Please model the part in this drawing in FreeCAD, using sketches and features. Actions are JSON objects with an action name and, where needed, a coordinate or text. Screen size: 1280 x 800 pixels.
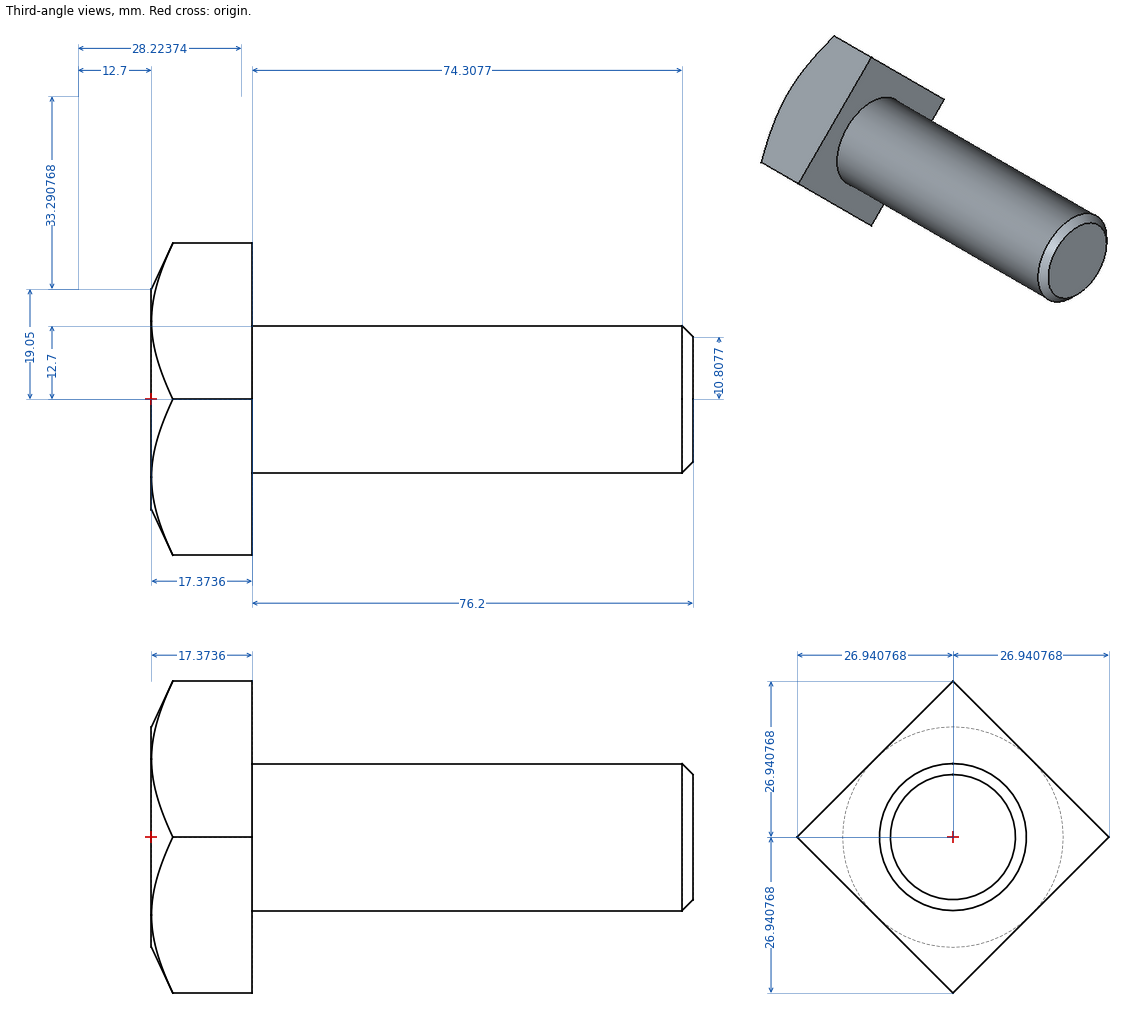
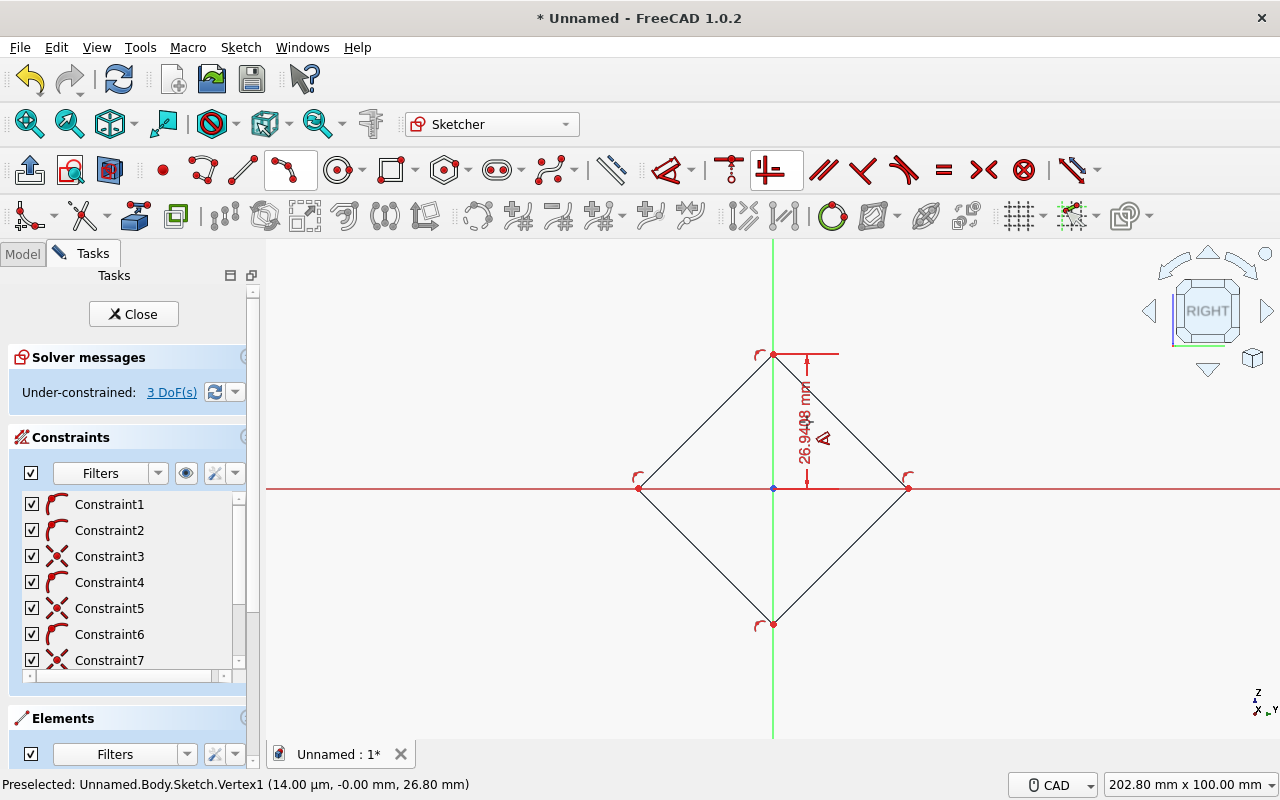
{"action": "left_click", "coordinate": [638, 489]}
{"action": "left_click", "coordinate": [705, 523]}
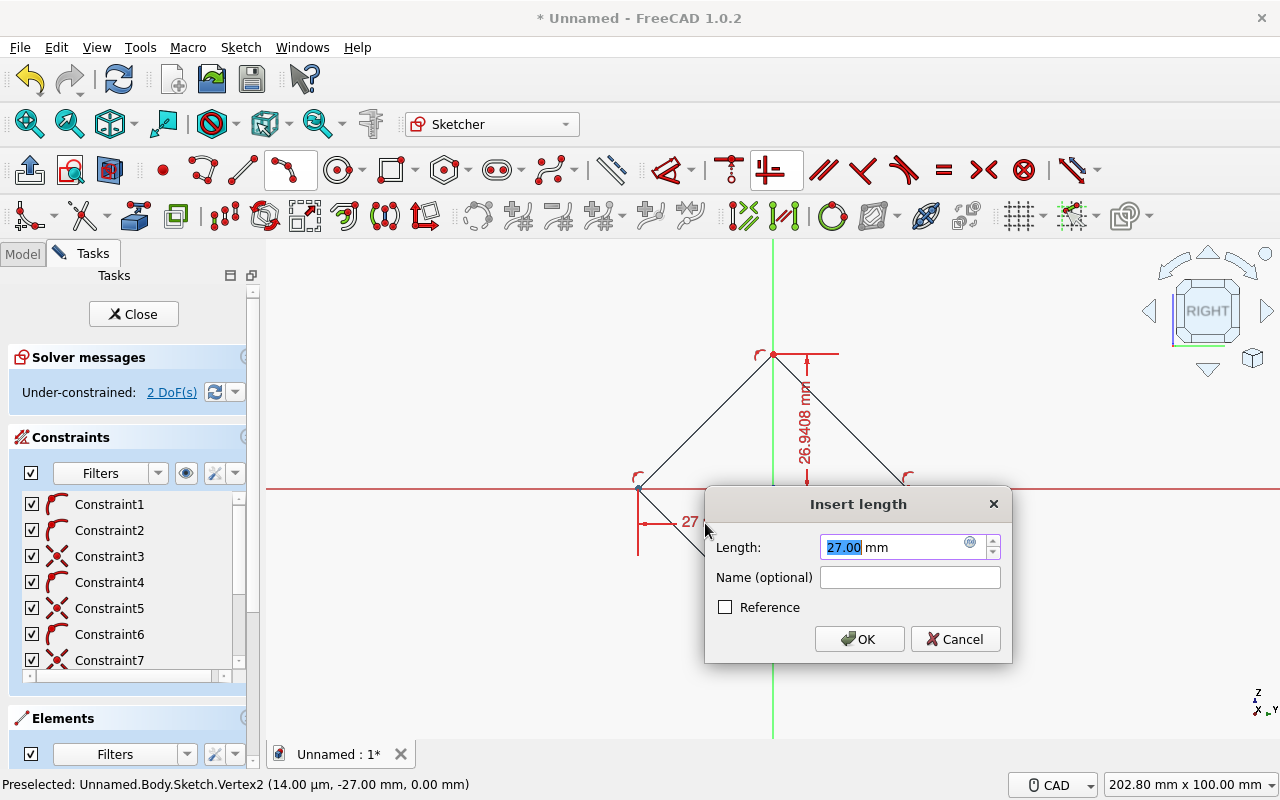
{"action": "type", "text": "26.940768"}
{"action": "key", "text": "Return"}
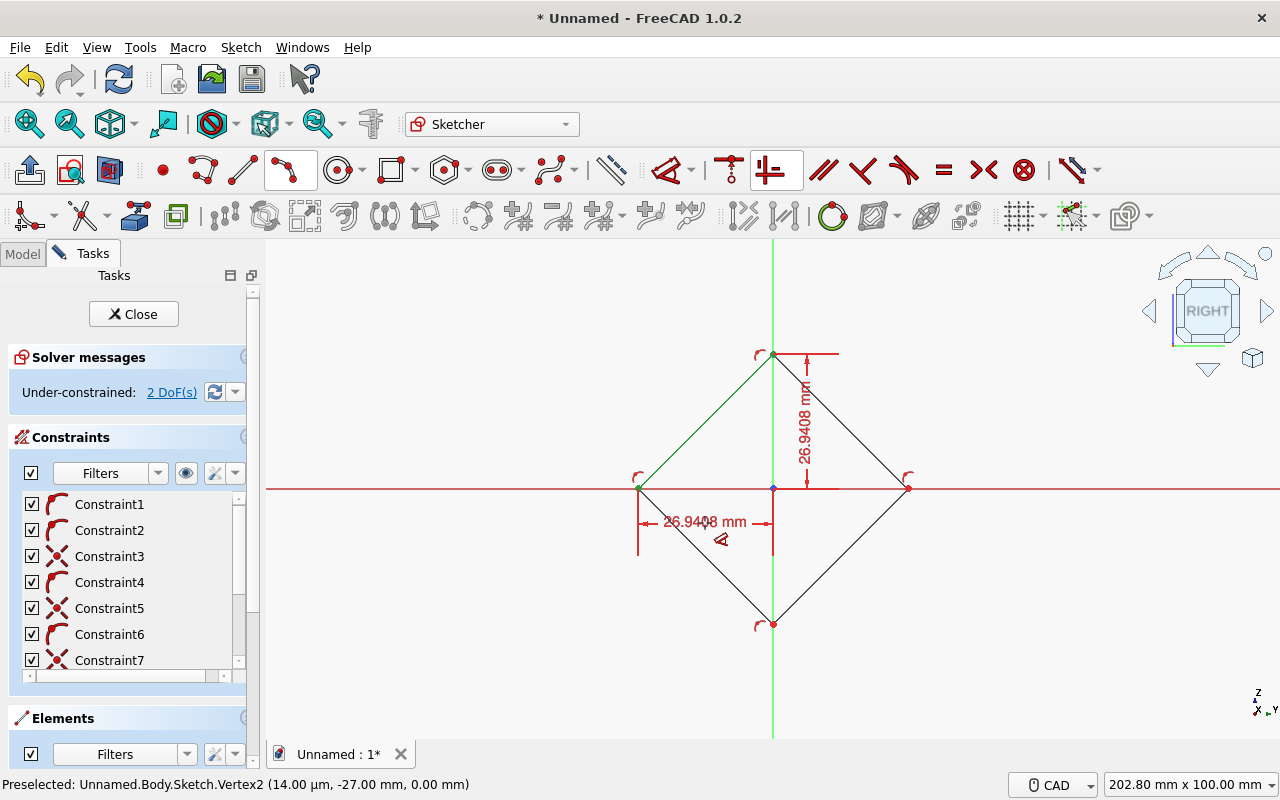
{"action": "left_click", "coordinate": [773, 625]}
{"action": "left_click", "coordinate": [807, 557]}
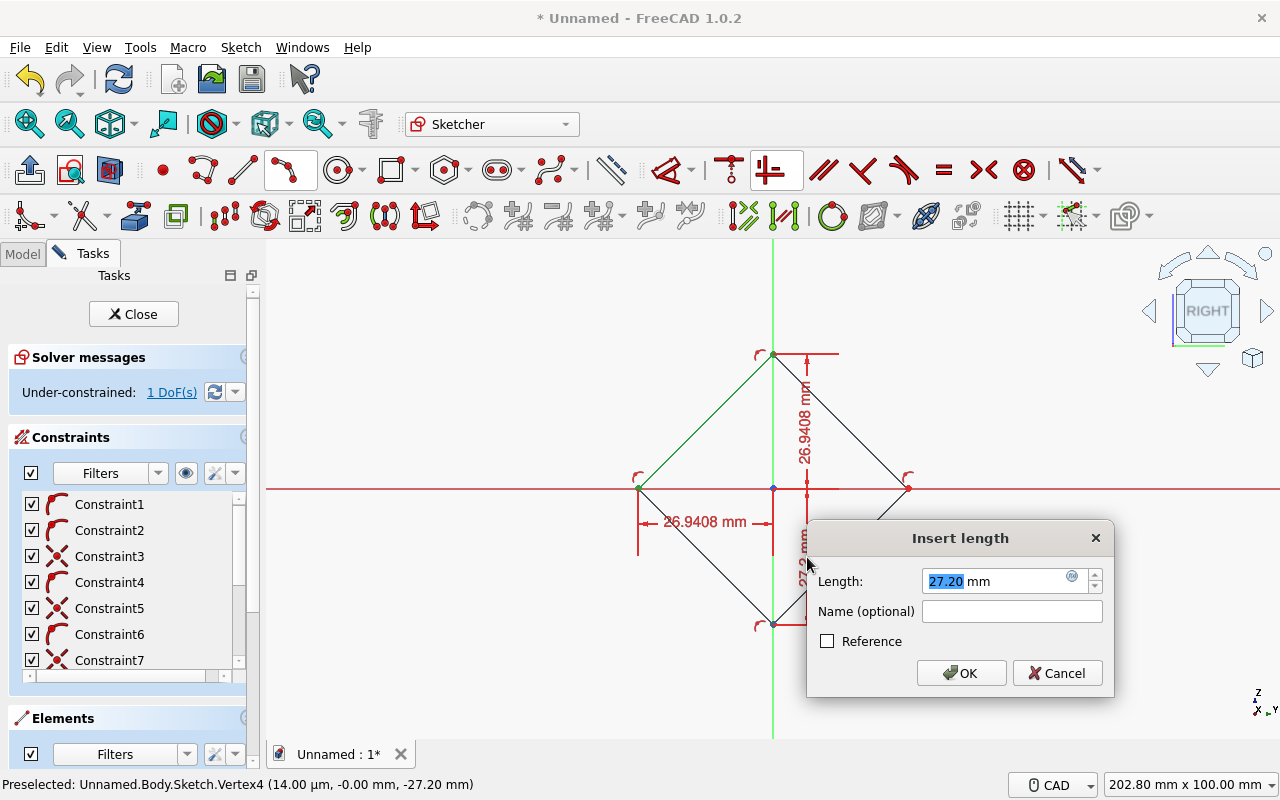
{"action": "type", "text": "26.940768"}
{"action": "key", "text": "Return"}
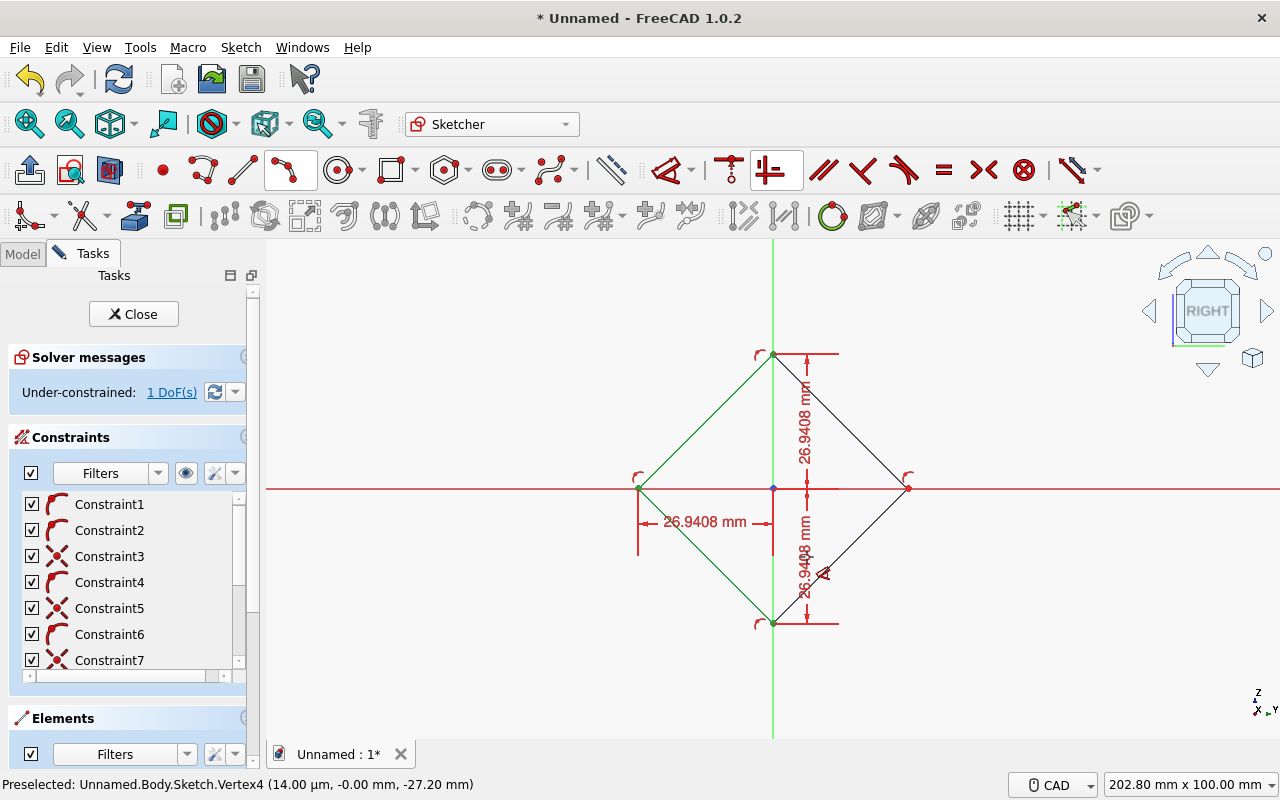
{"action": "left_click", "coordinate": [908, 489]}
{"action": "left_click", "coordinate": [840, 523]}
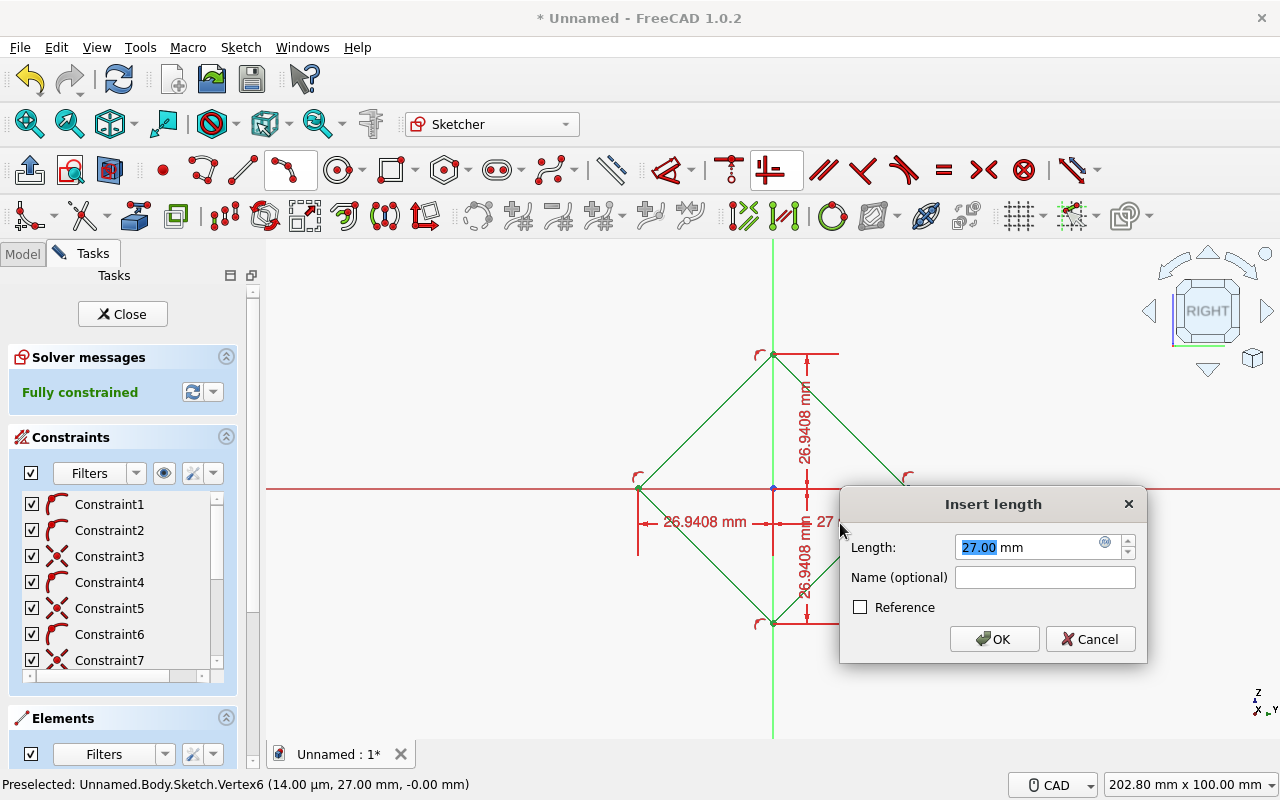
{"action": "type", "text": "26.940768"}
{"action": "key", "text": "Return"}
{"action": "key", "text": "Escape"}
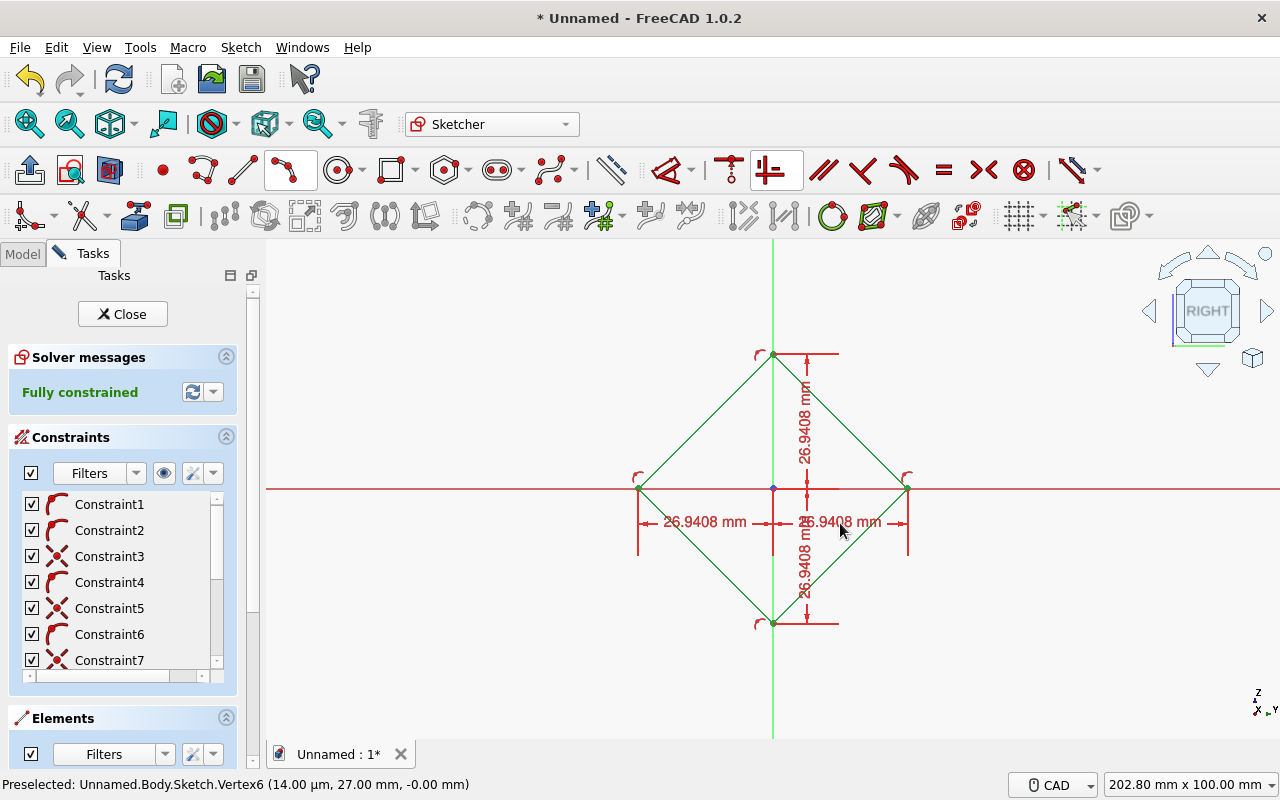
{"action": "left_click", "coordinate": [123, 314]}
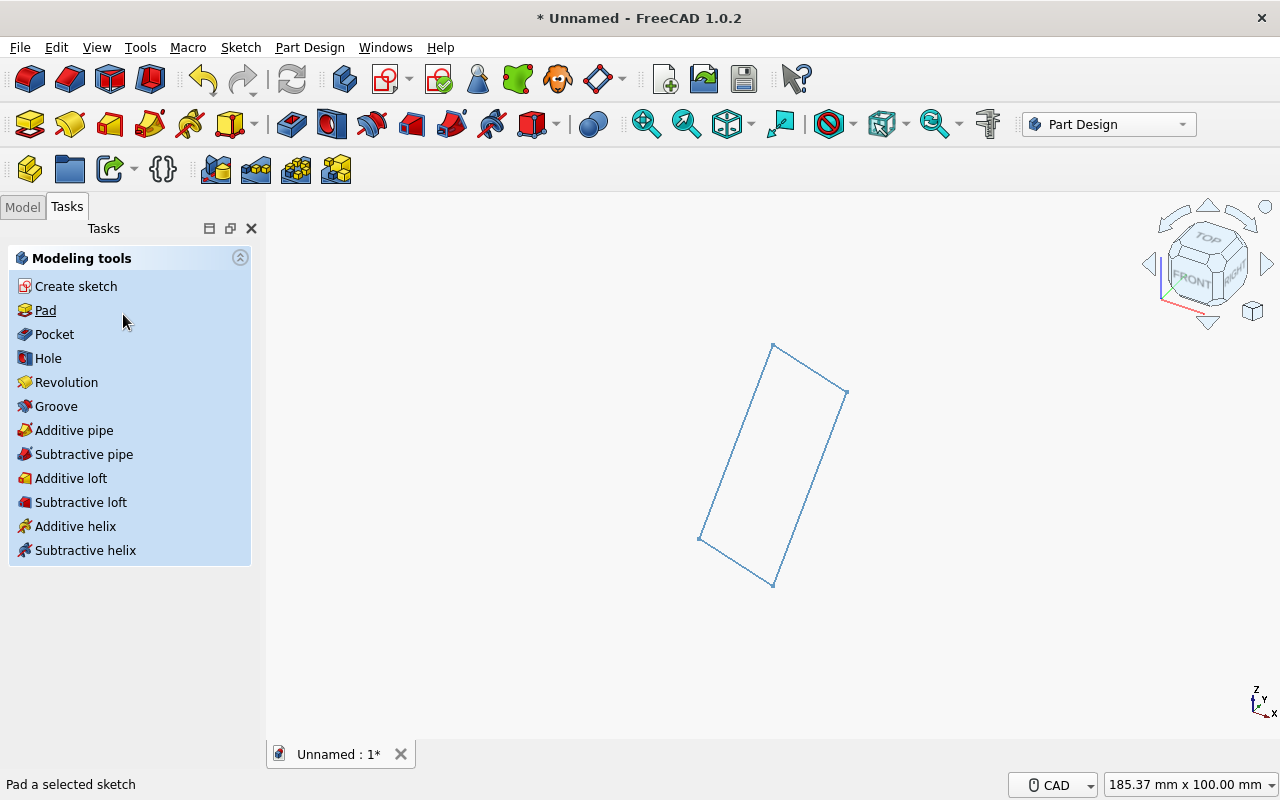
{"action": "left_click", "coordinate": [30, 124]}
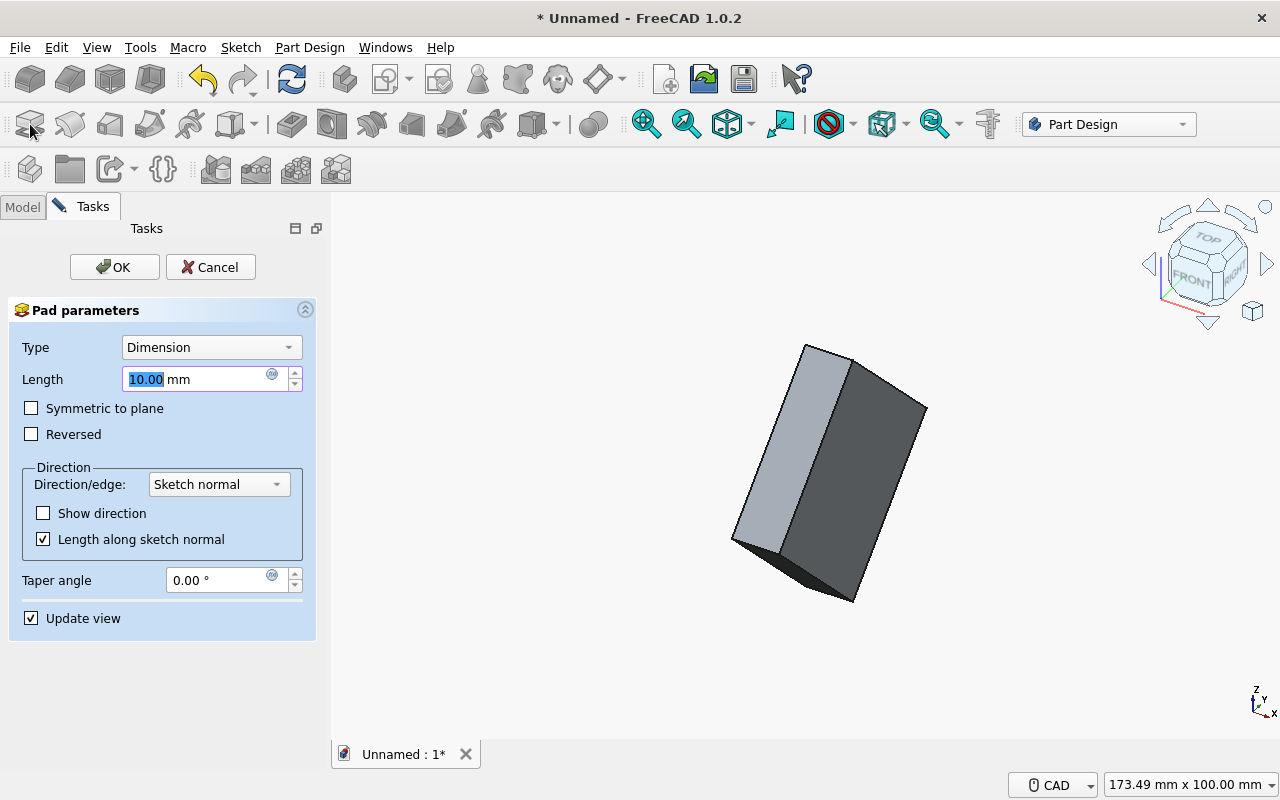
{"action": "type", "text": "17.3736"}
{"action": "key", "text": "Tab"}